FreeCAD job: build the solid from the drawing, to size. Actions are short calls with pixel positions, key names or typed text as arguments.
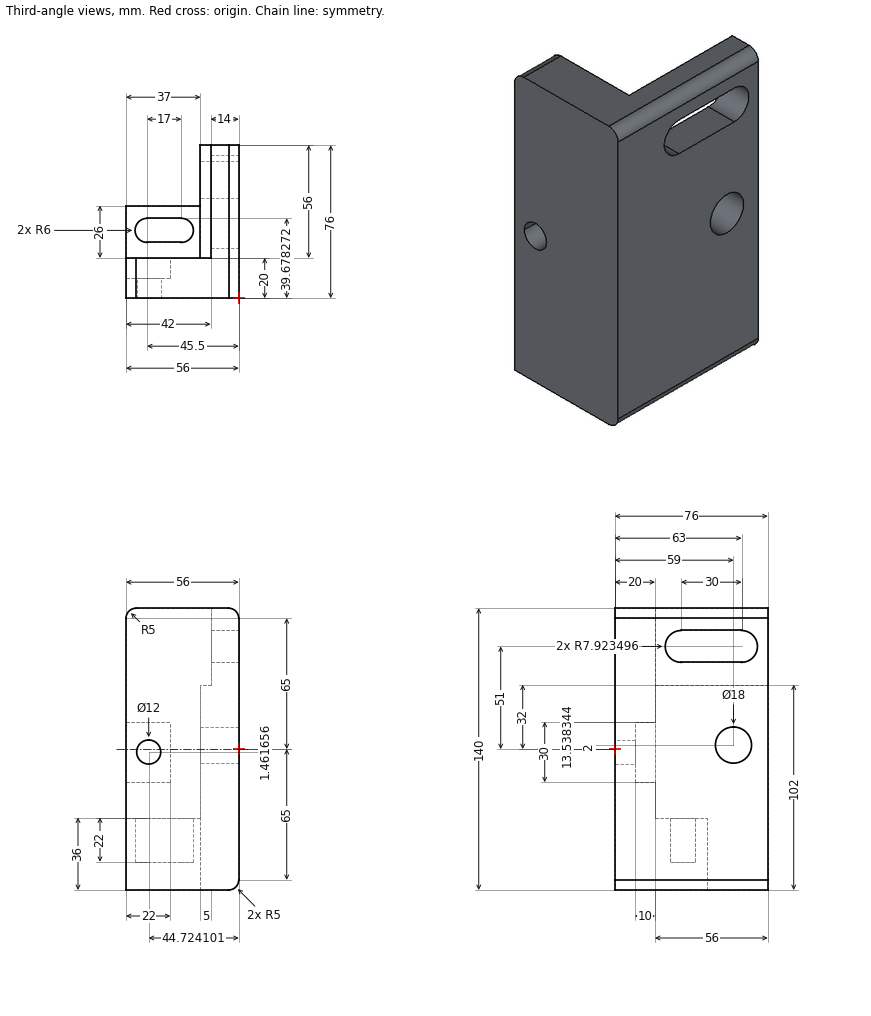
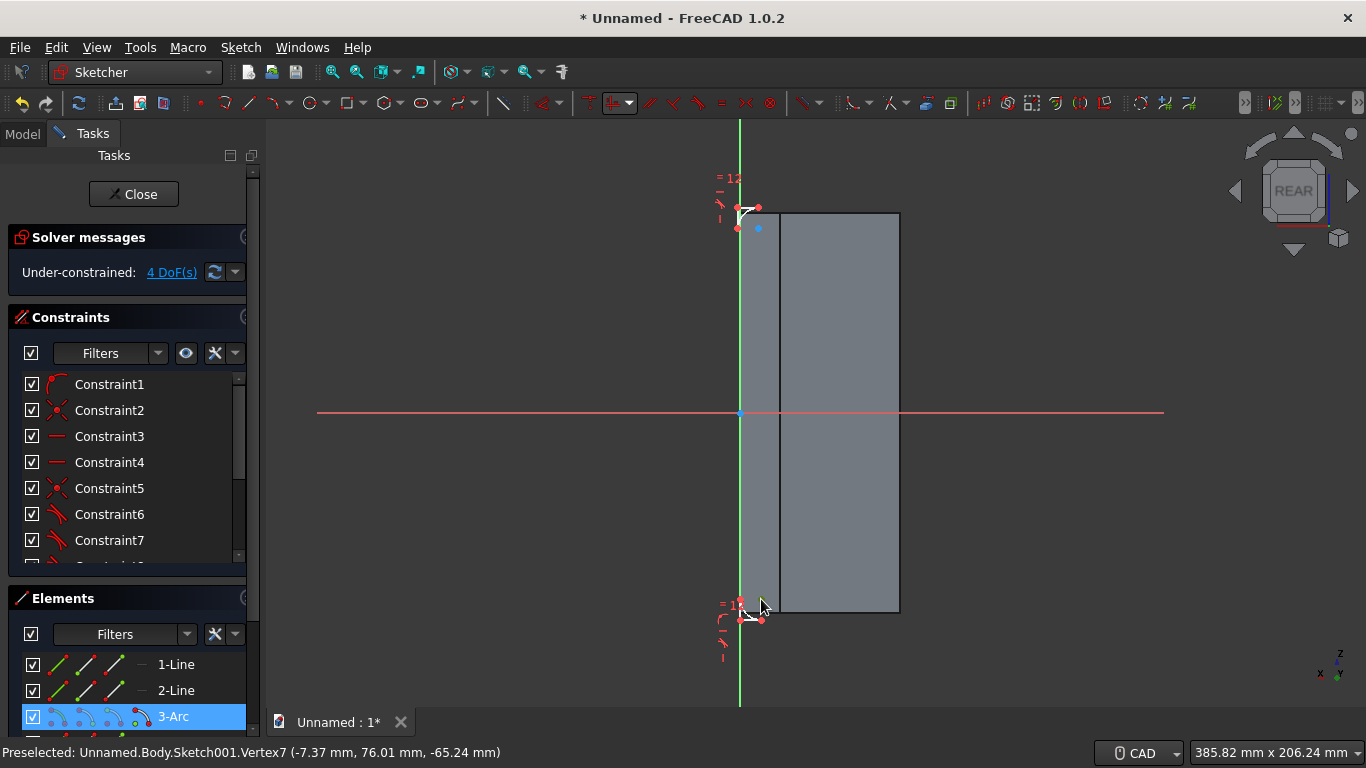
click(759, 229)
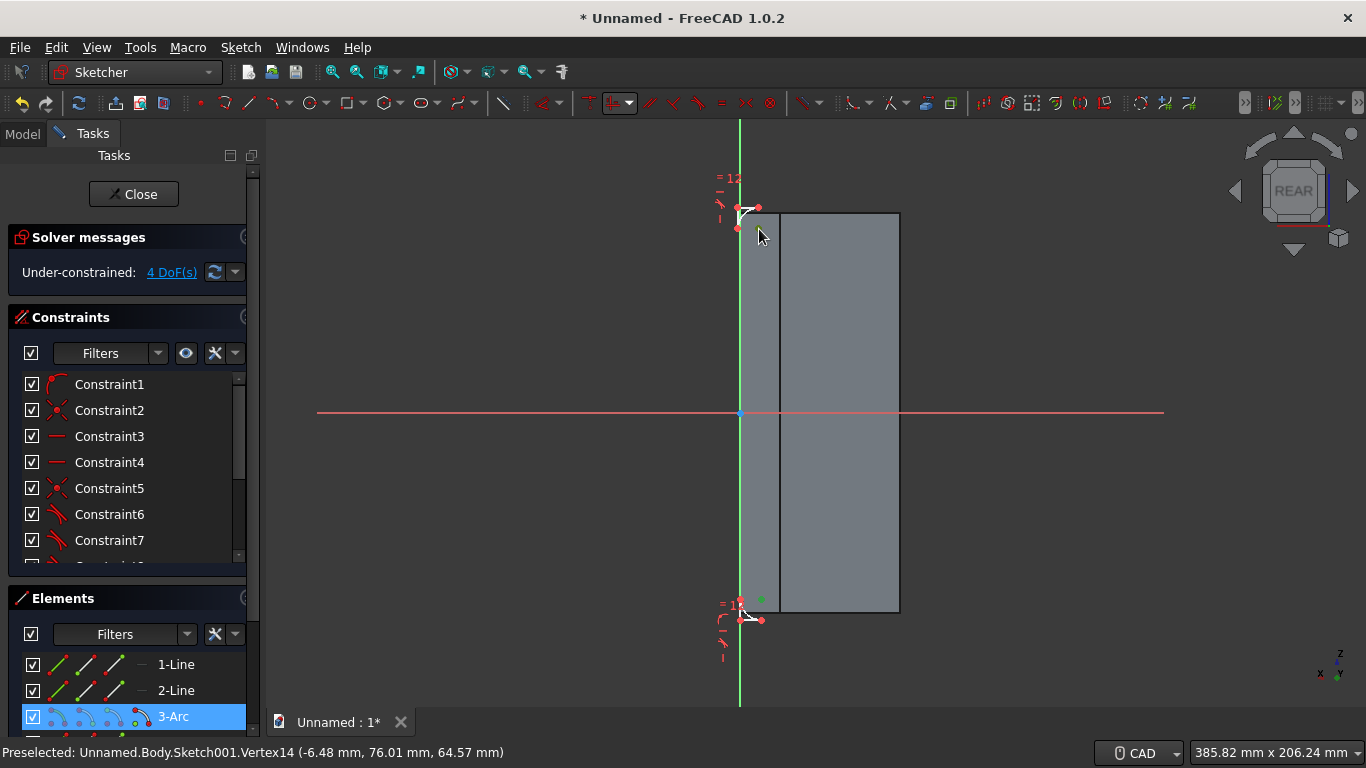
click(359, 413)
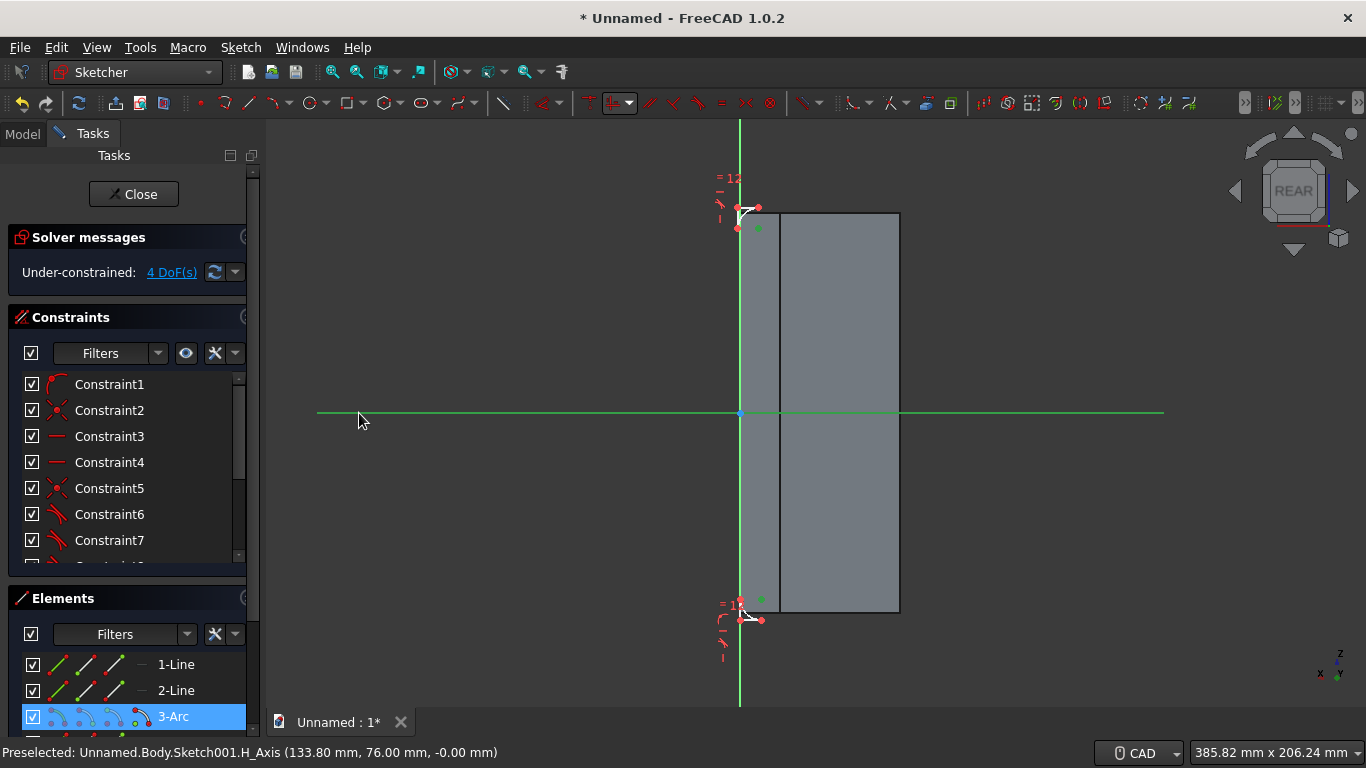
key(s)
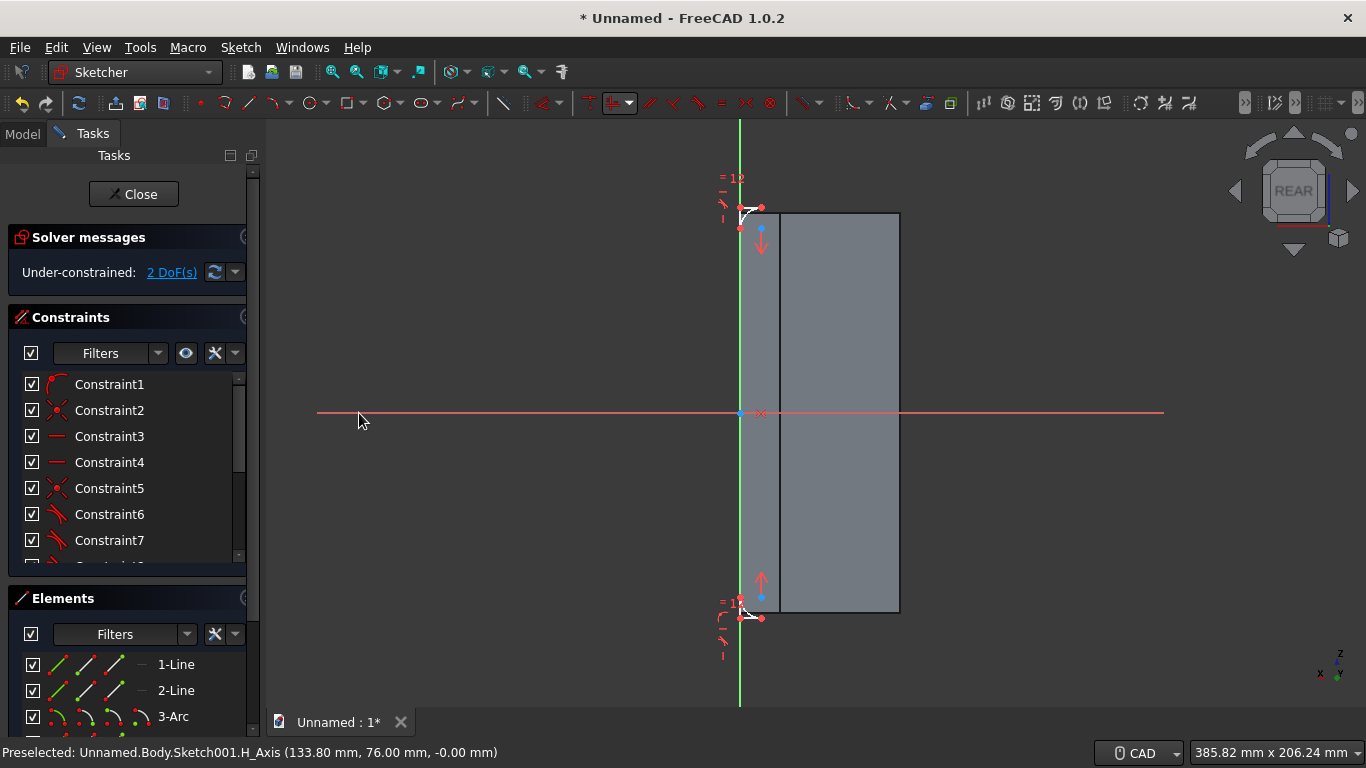
click(542, 104)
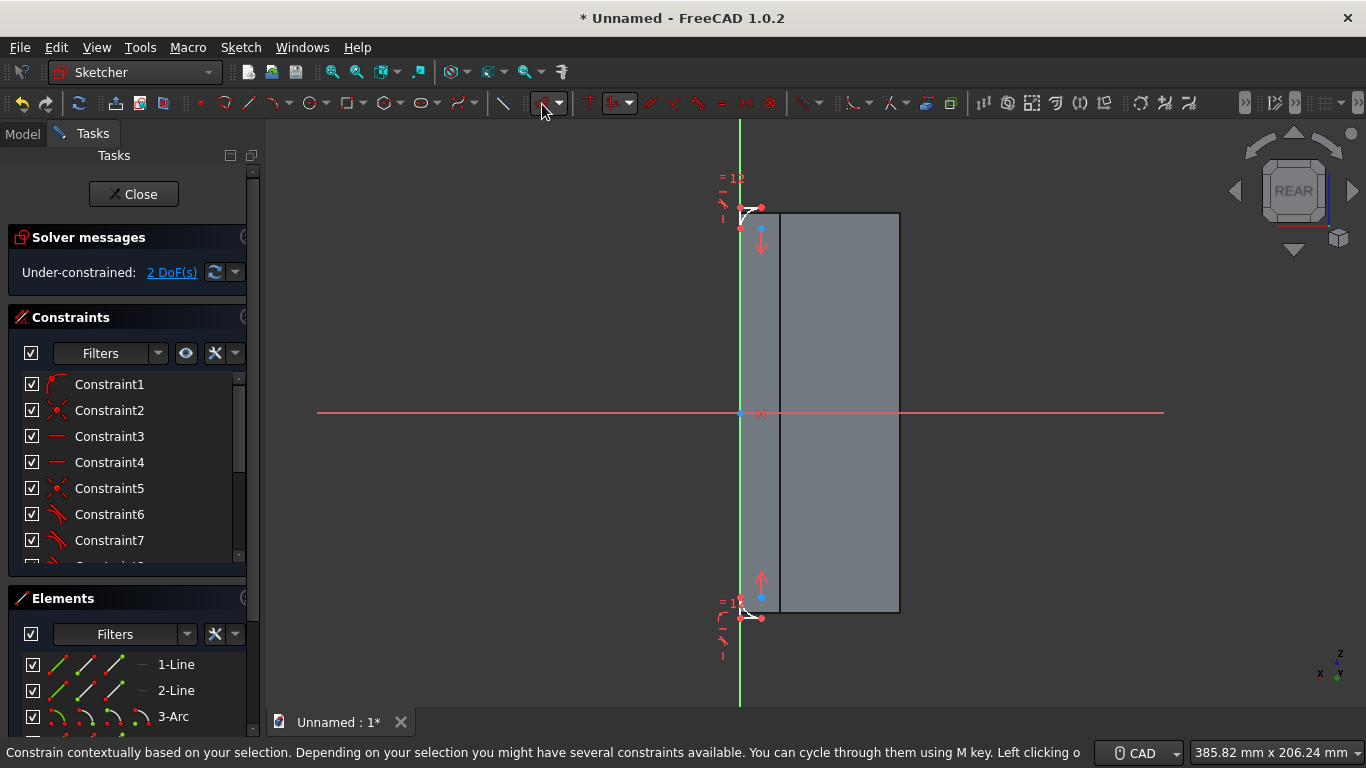
scroll(747, 612, up, 6)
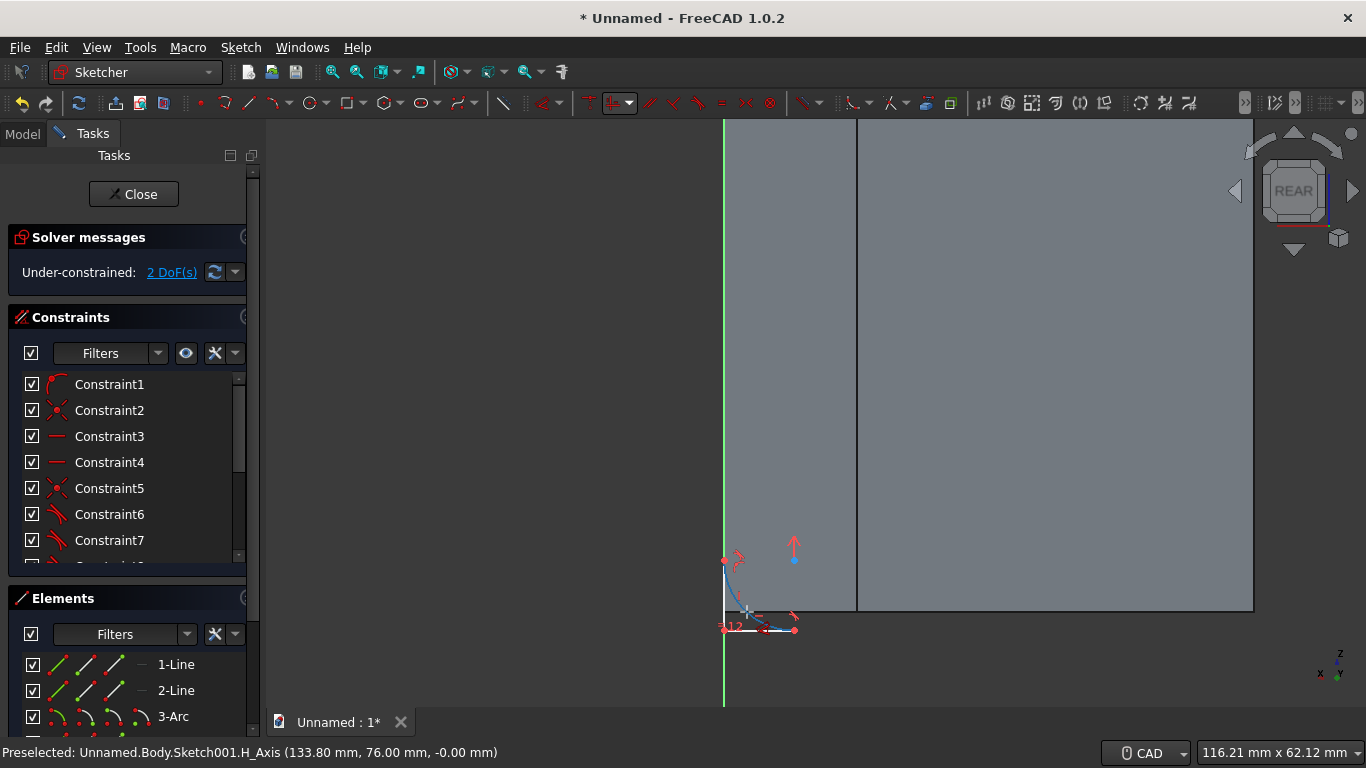
click(745, 610)
click(697, 589)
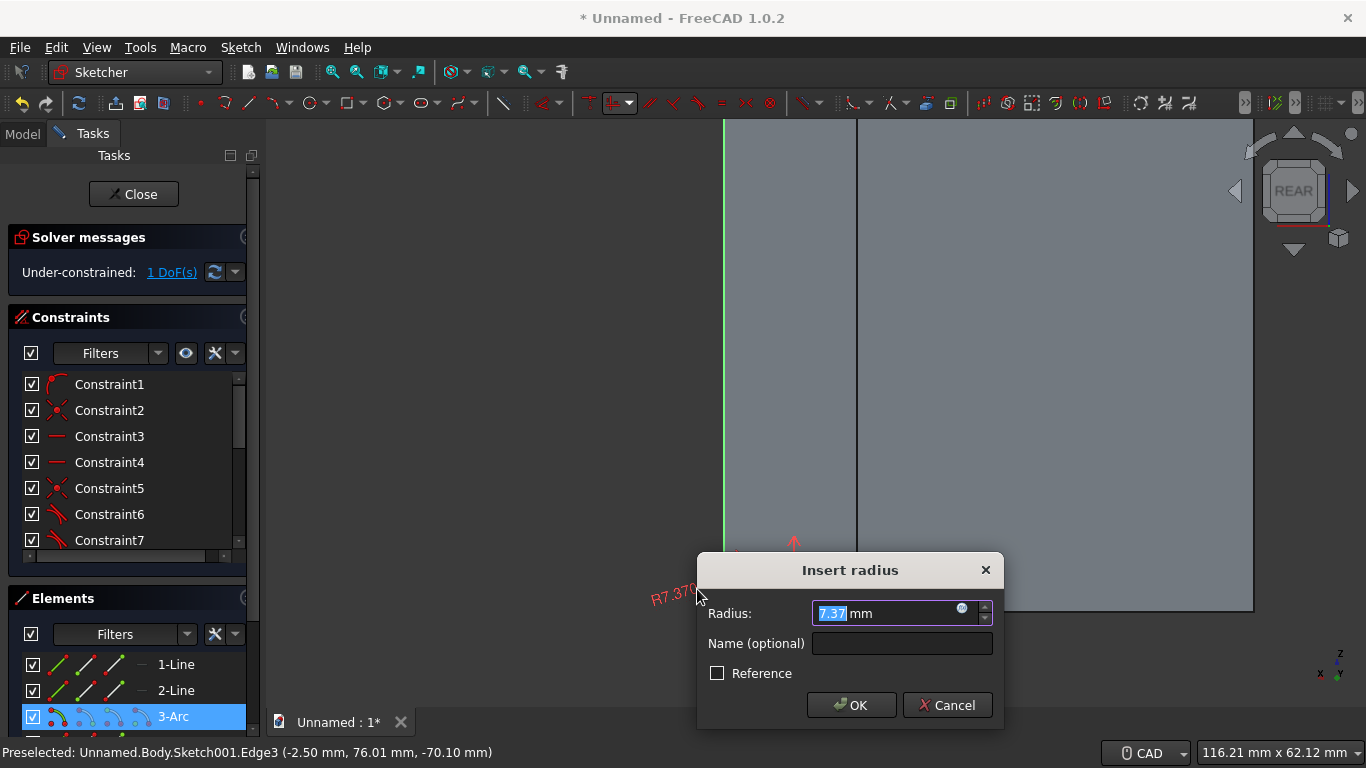
text(5)
key(Return)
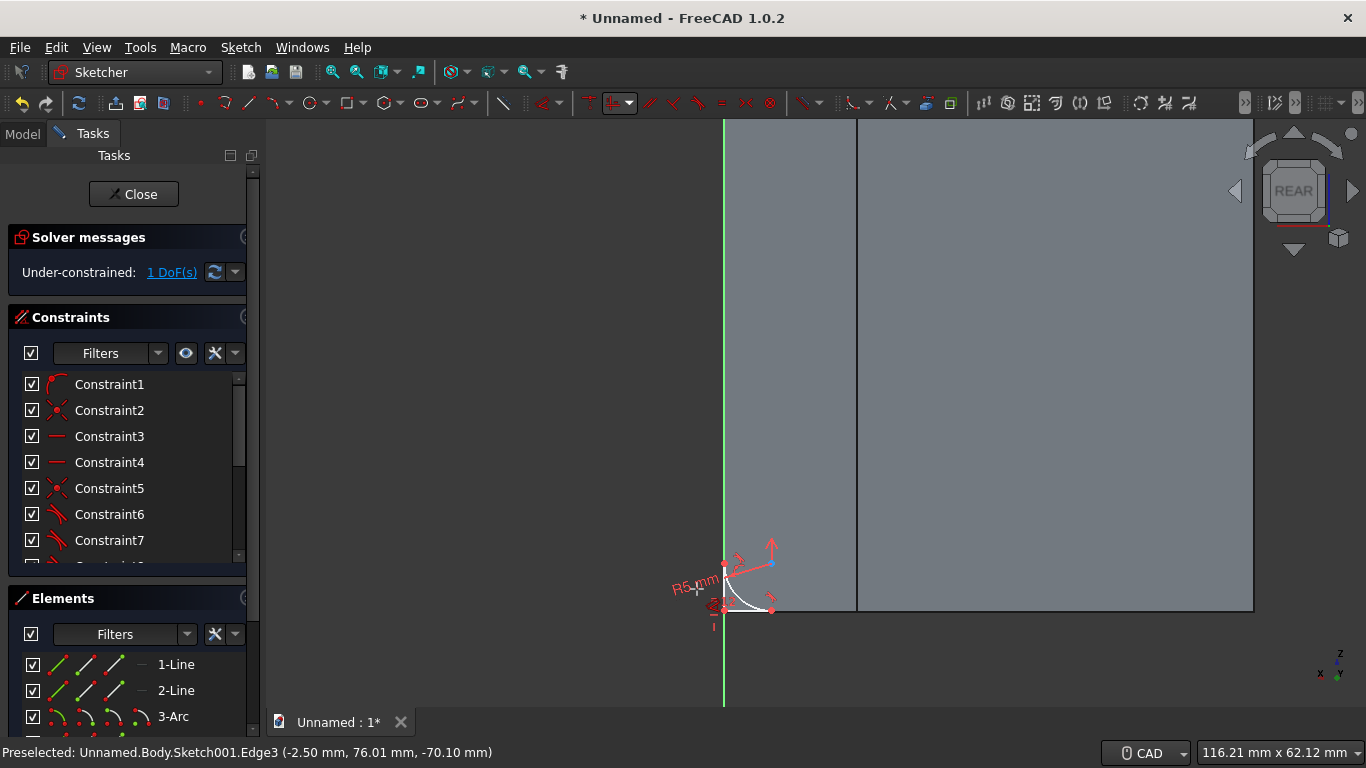
click(724, 564)
click(690, 355)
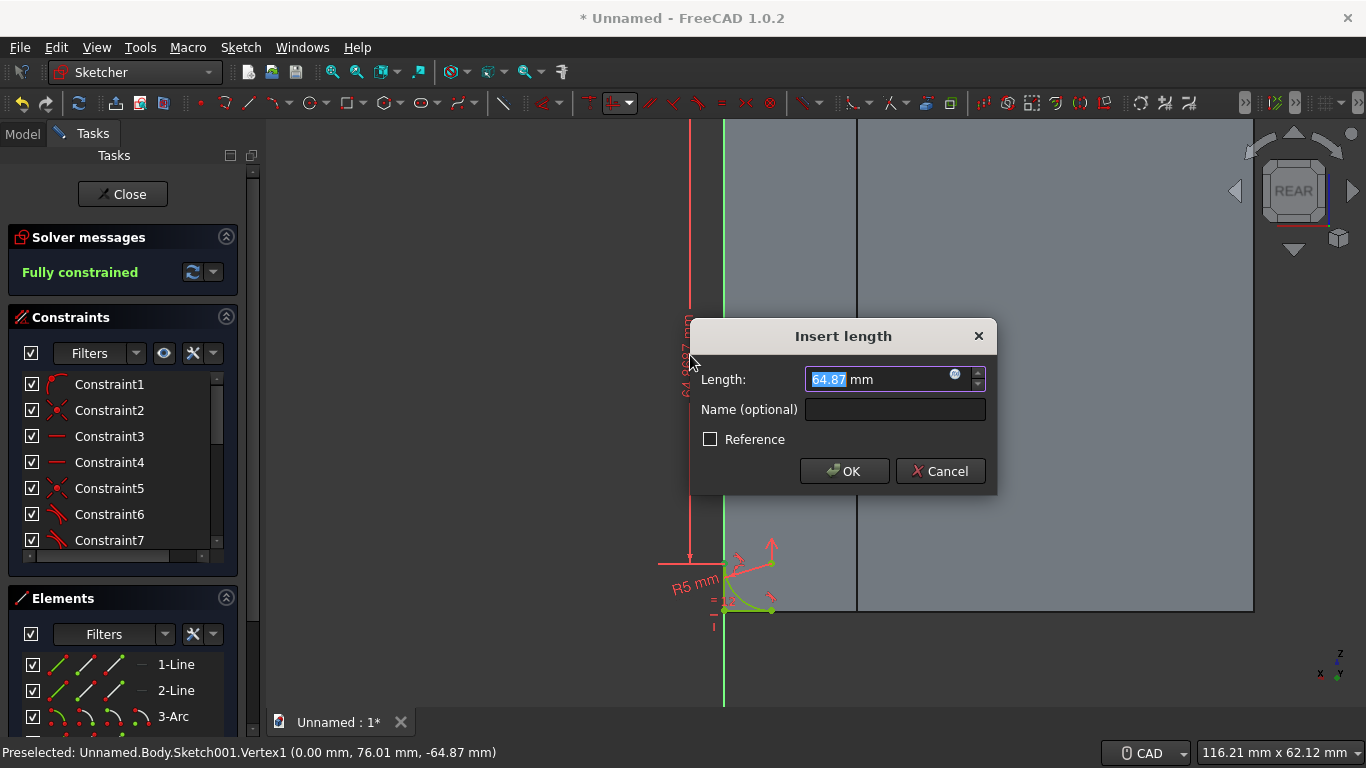
text(65)
key(Return)
key(Escape)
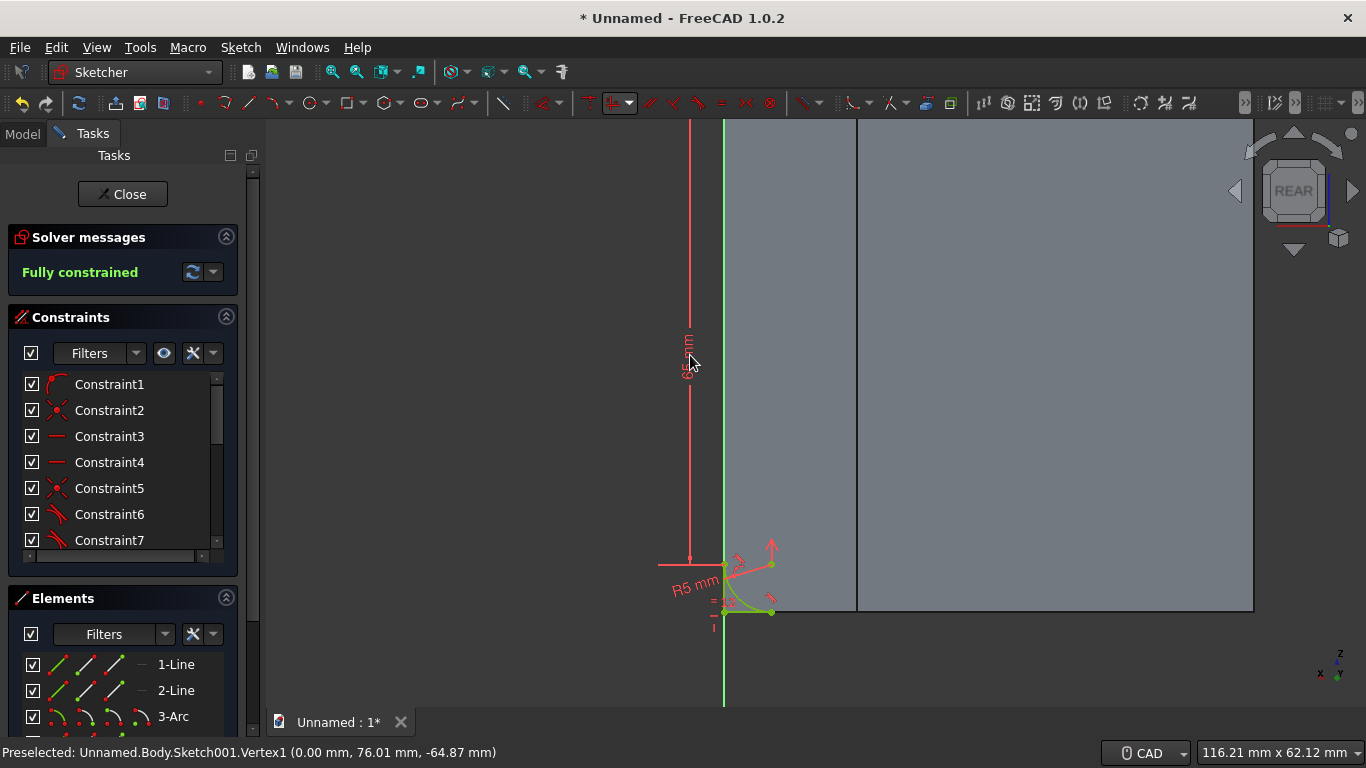
click(123, 194)